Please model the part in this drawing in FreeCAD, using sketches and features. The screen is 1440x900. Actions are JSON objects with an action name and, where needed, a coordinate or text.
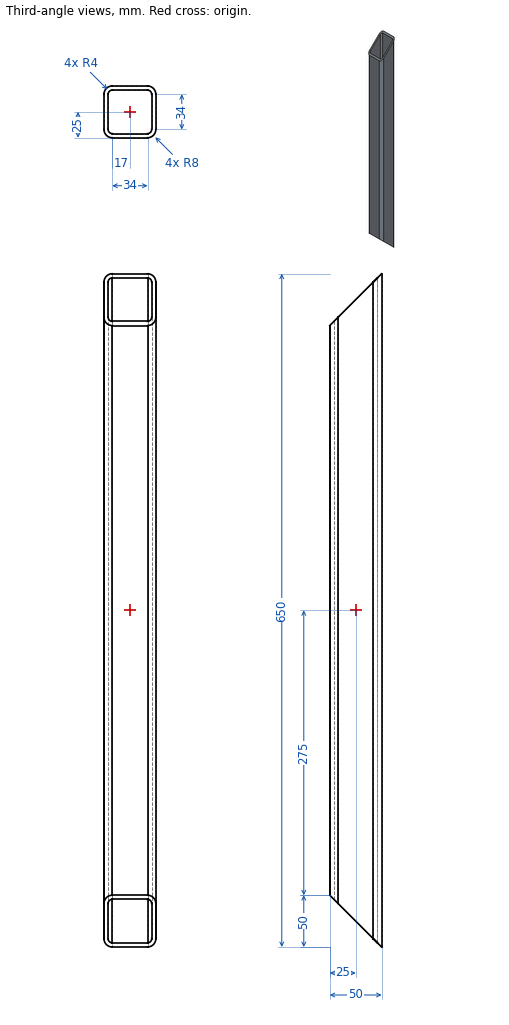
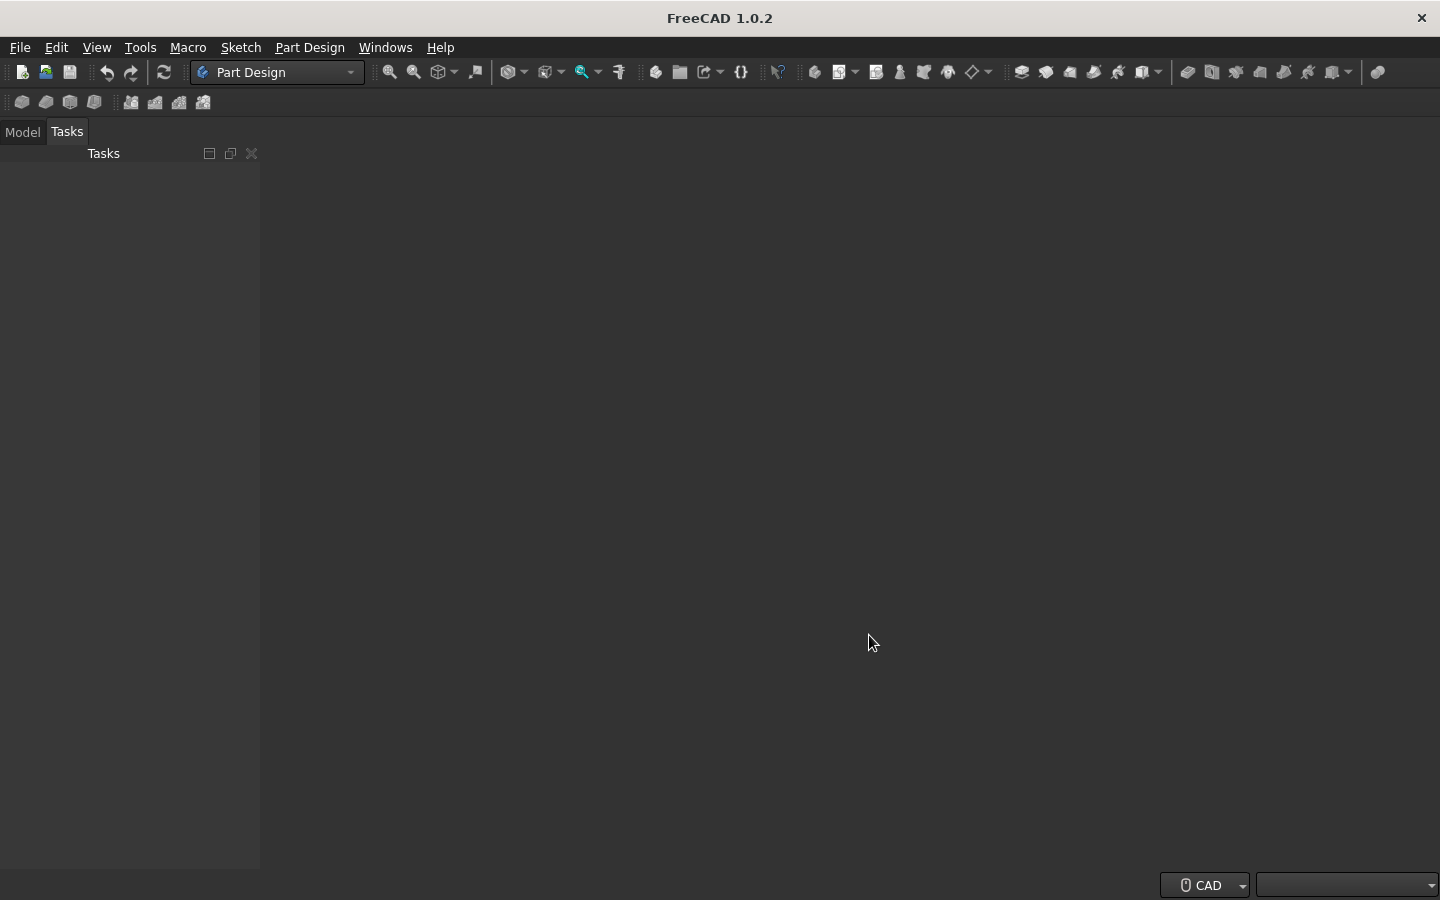
{"action": "left_click", "coordinate": [22, 72]}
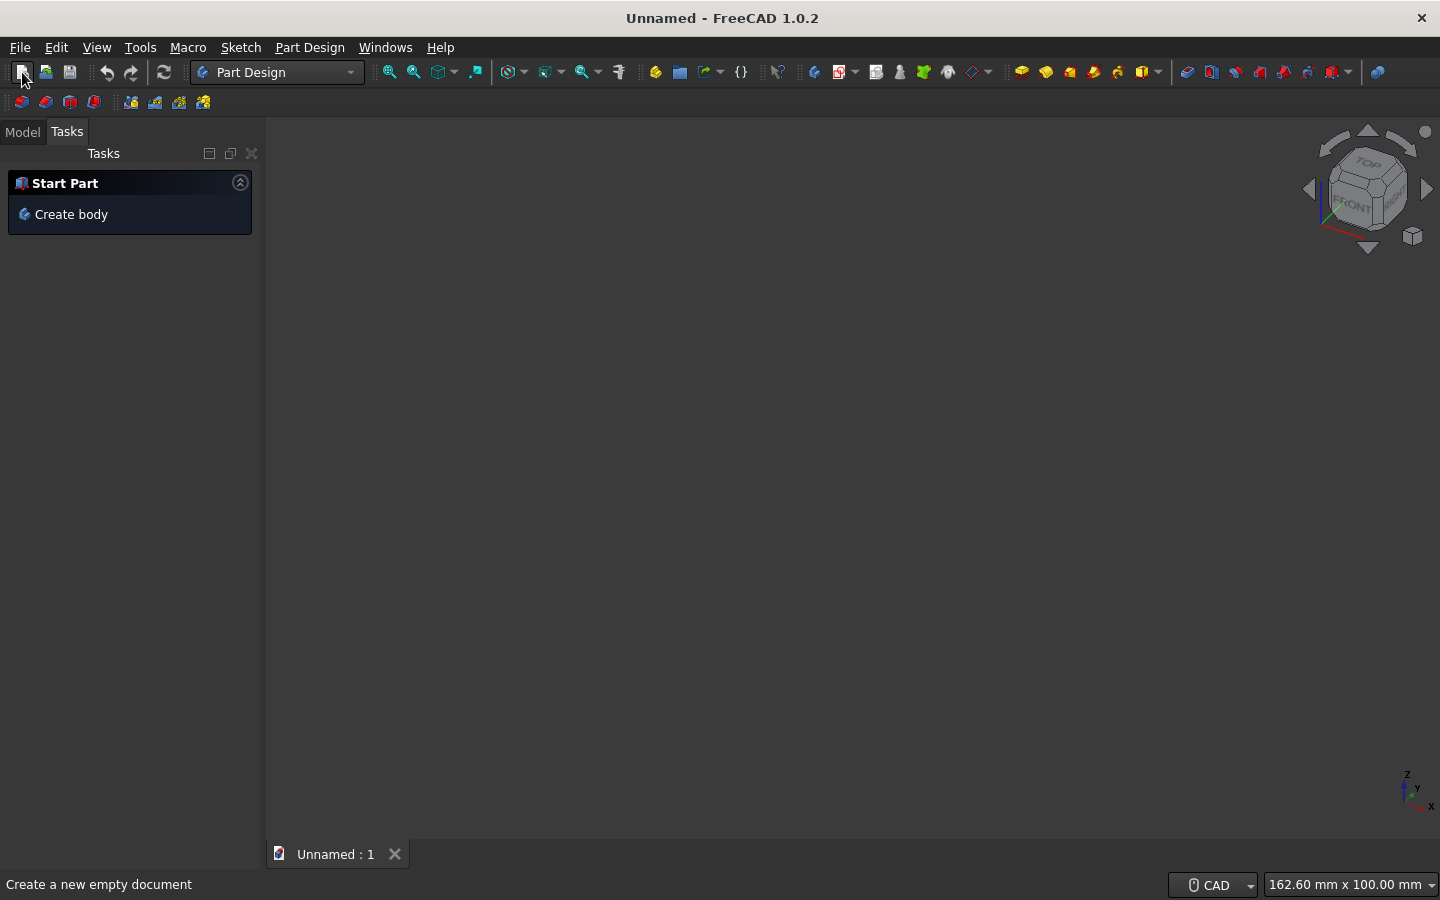
{"action": "left_click", "coordinate": [840, 72]}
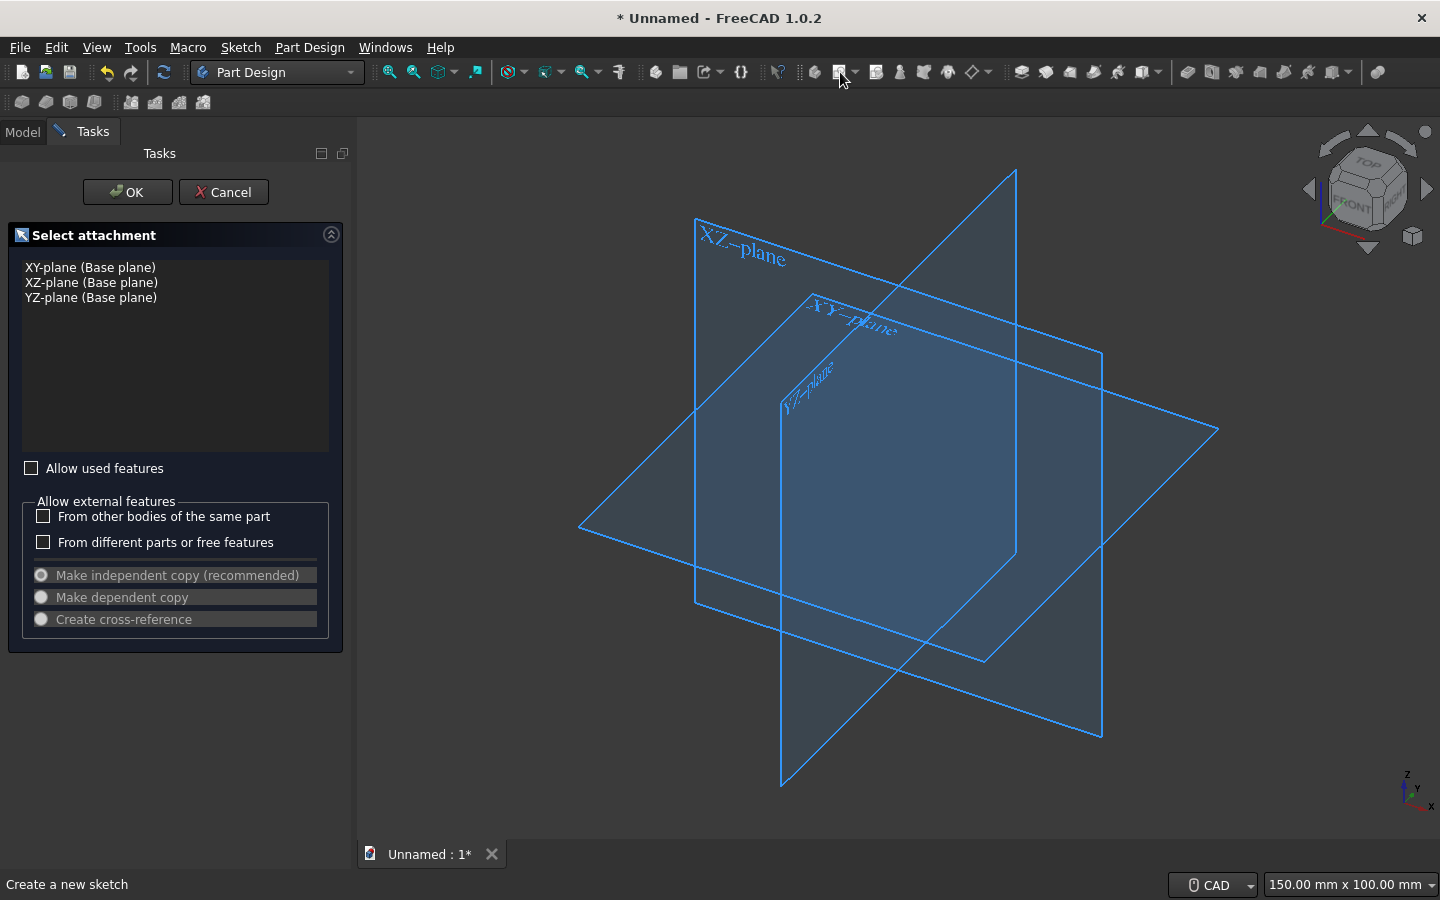
{"action": "left_click", "coordinate": [82, 268]}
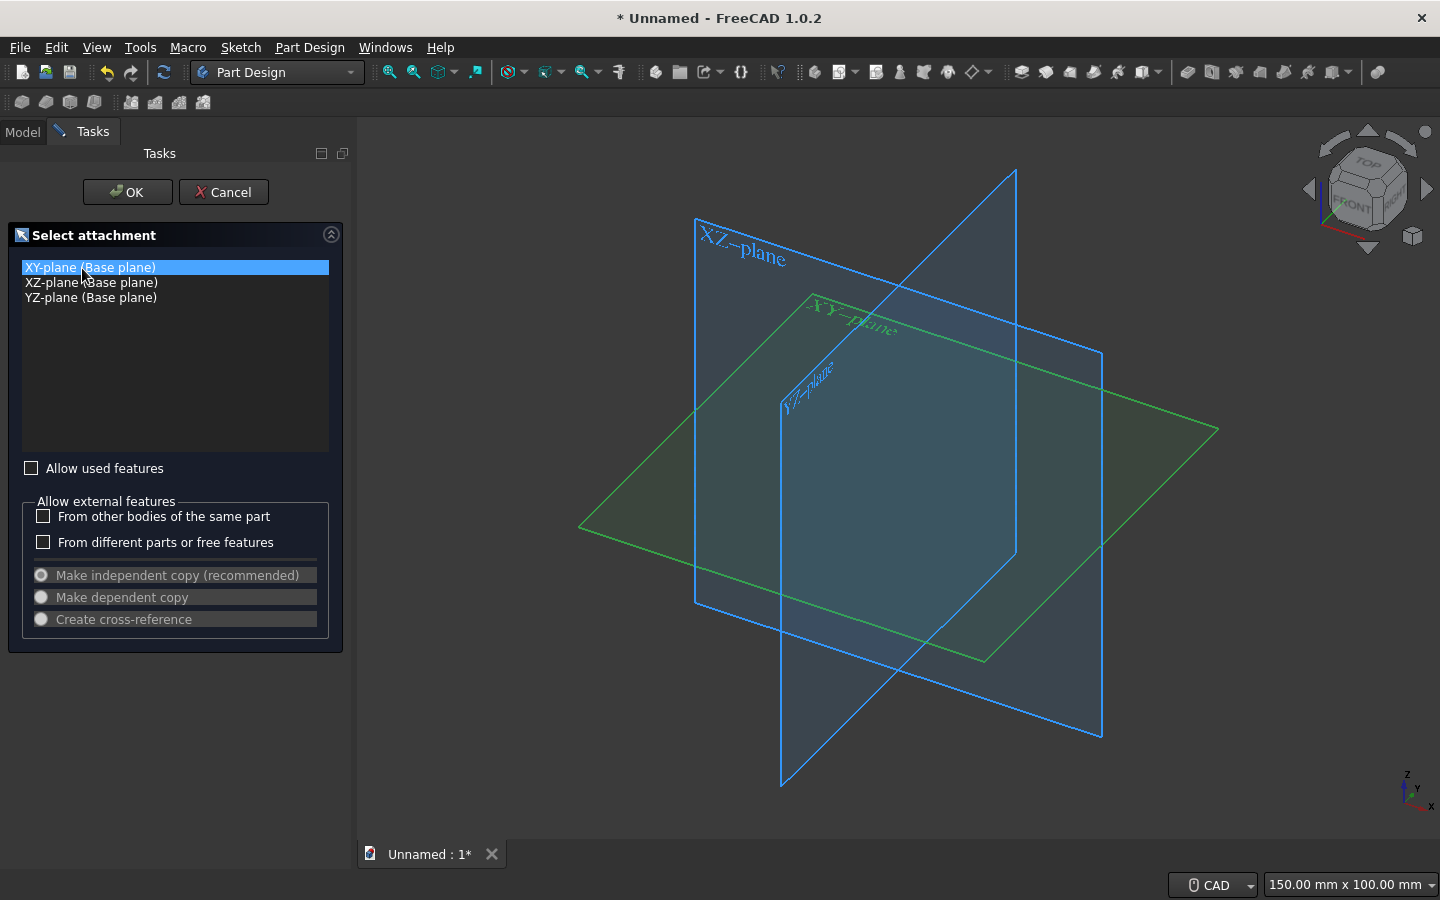
{"action": "left_click", "coordinate": [128, 192]}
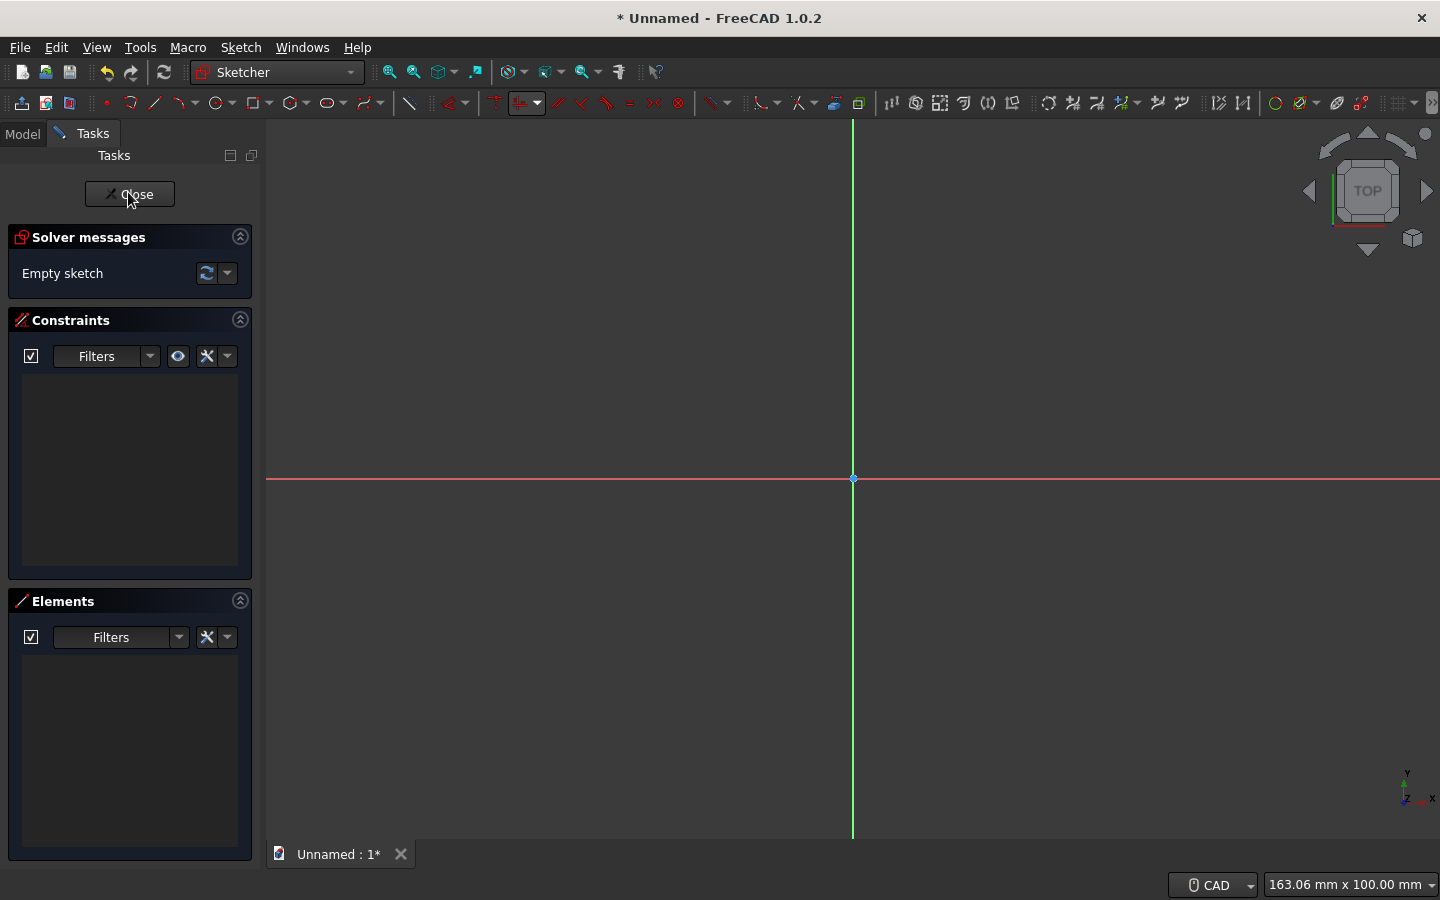
{"action": "left_click", "coordinate": [156, 104]}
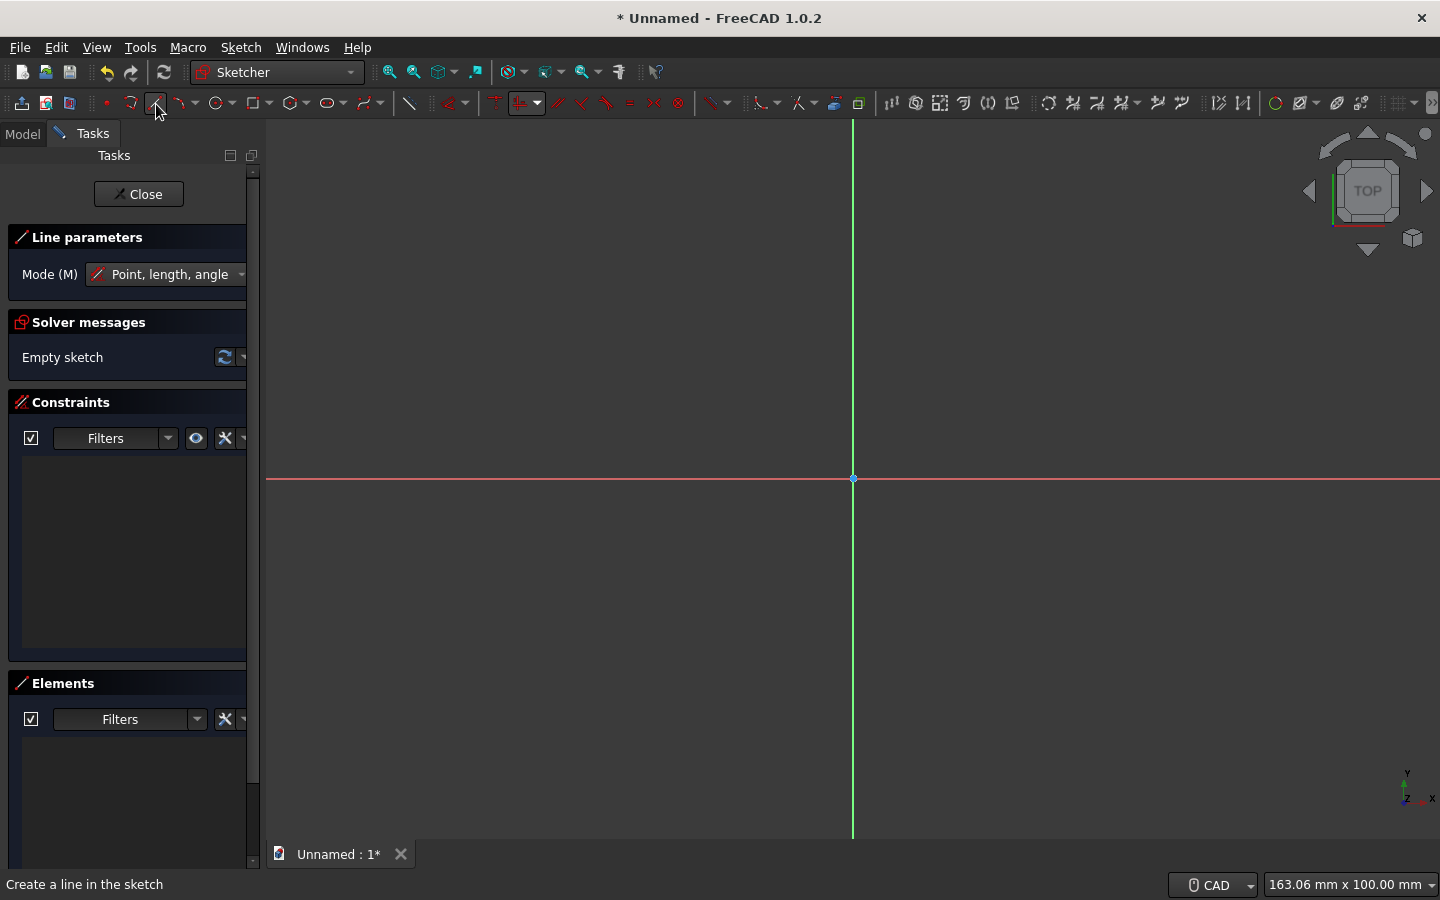
{"action": "left_click", "coordinate": [731, 659]}
{"action": "left_click", "coordinate": [975, 659]}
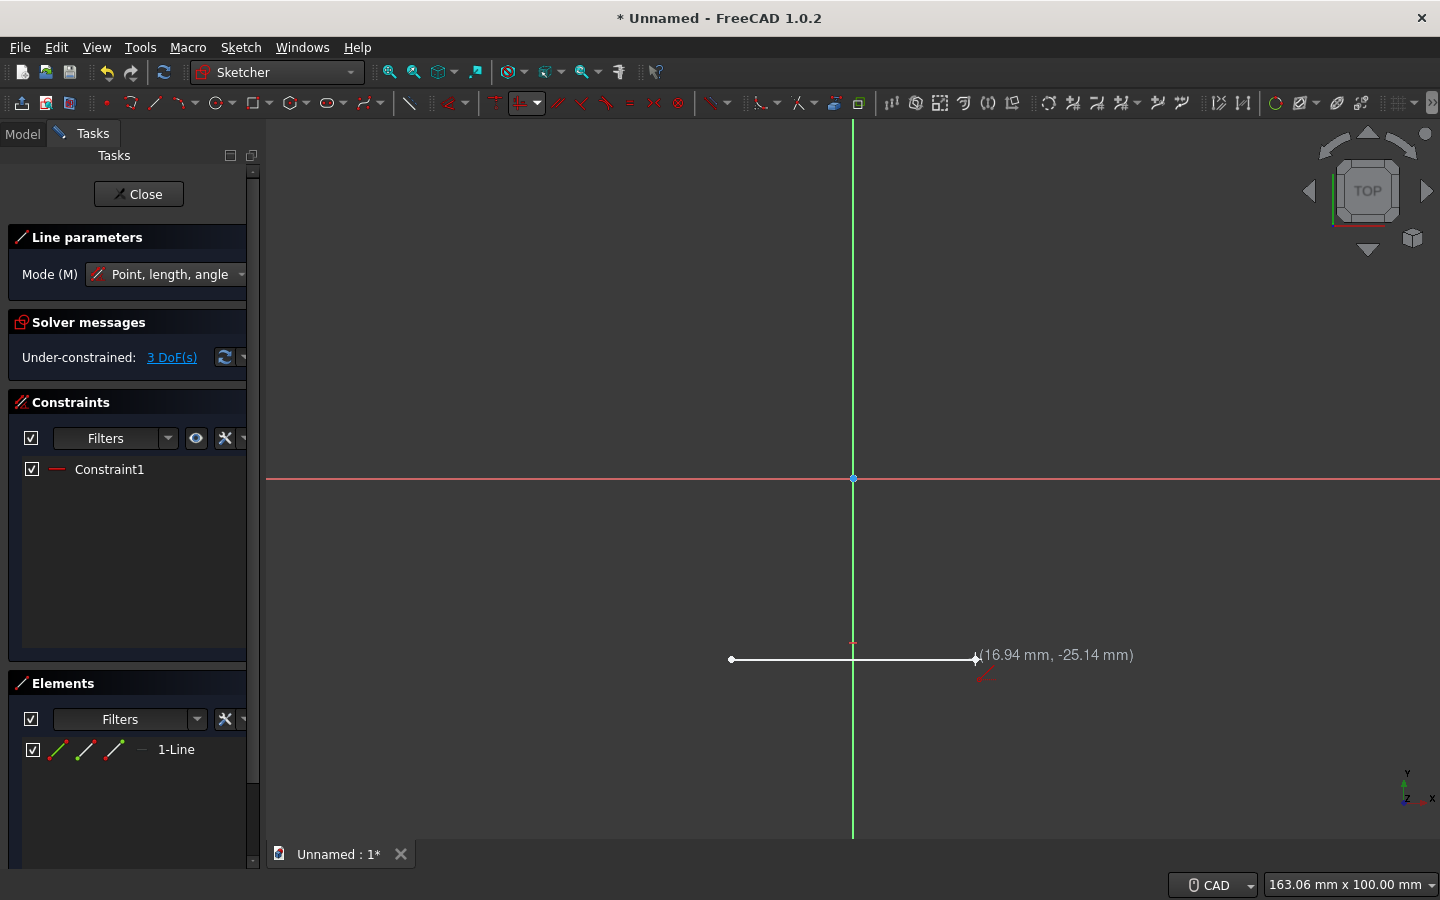
{"action": "left_click", "coordinate": [1033, 601]}
{"action": "left_click", "coordinate": [1033, 357]}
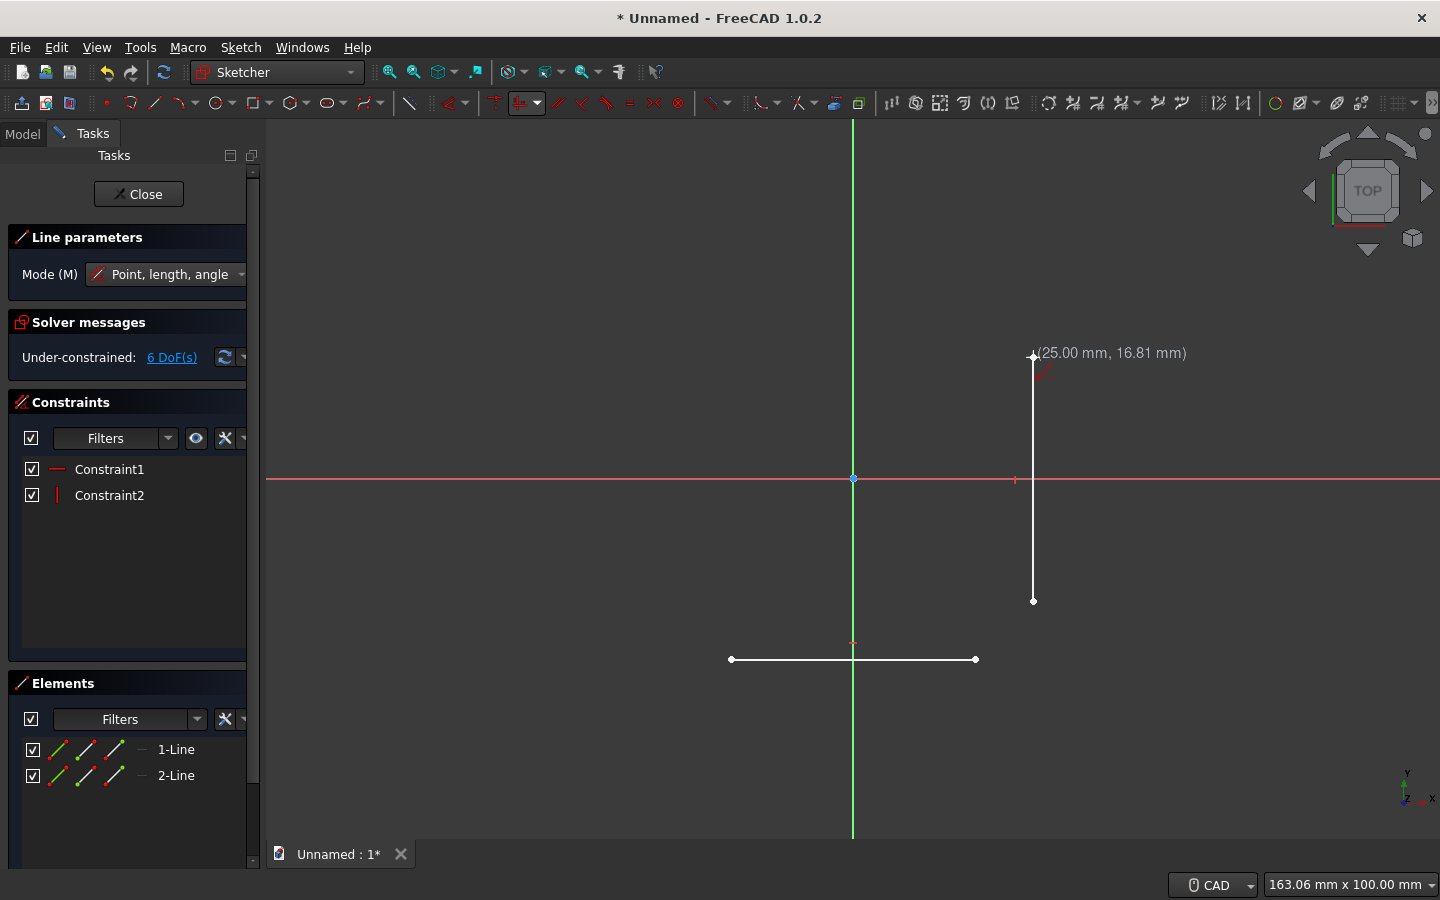
{"action": "left_click", "coordinate": [975, 299]}
{"action": "left_click", "coordinate": [731, 299]}